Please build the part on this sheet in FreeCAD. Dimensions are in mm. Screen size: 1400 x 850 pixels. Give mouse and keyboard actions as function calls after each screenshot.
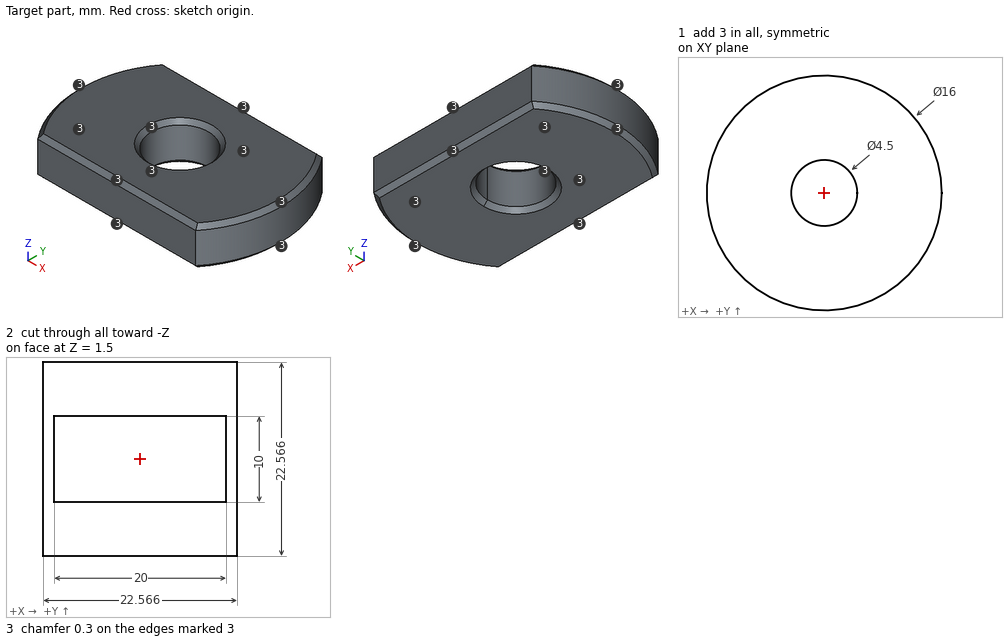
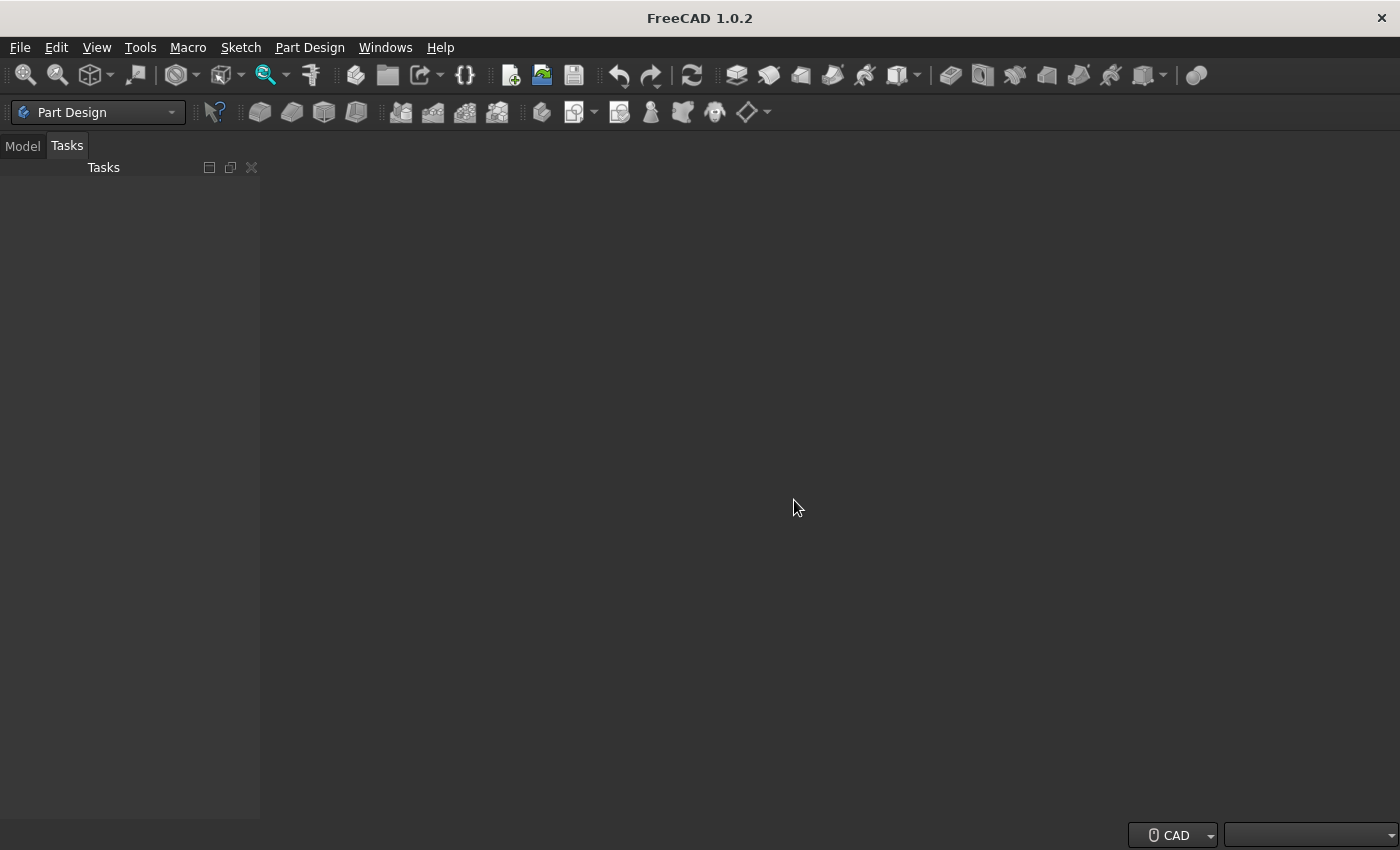
key(ctrl+n)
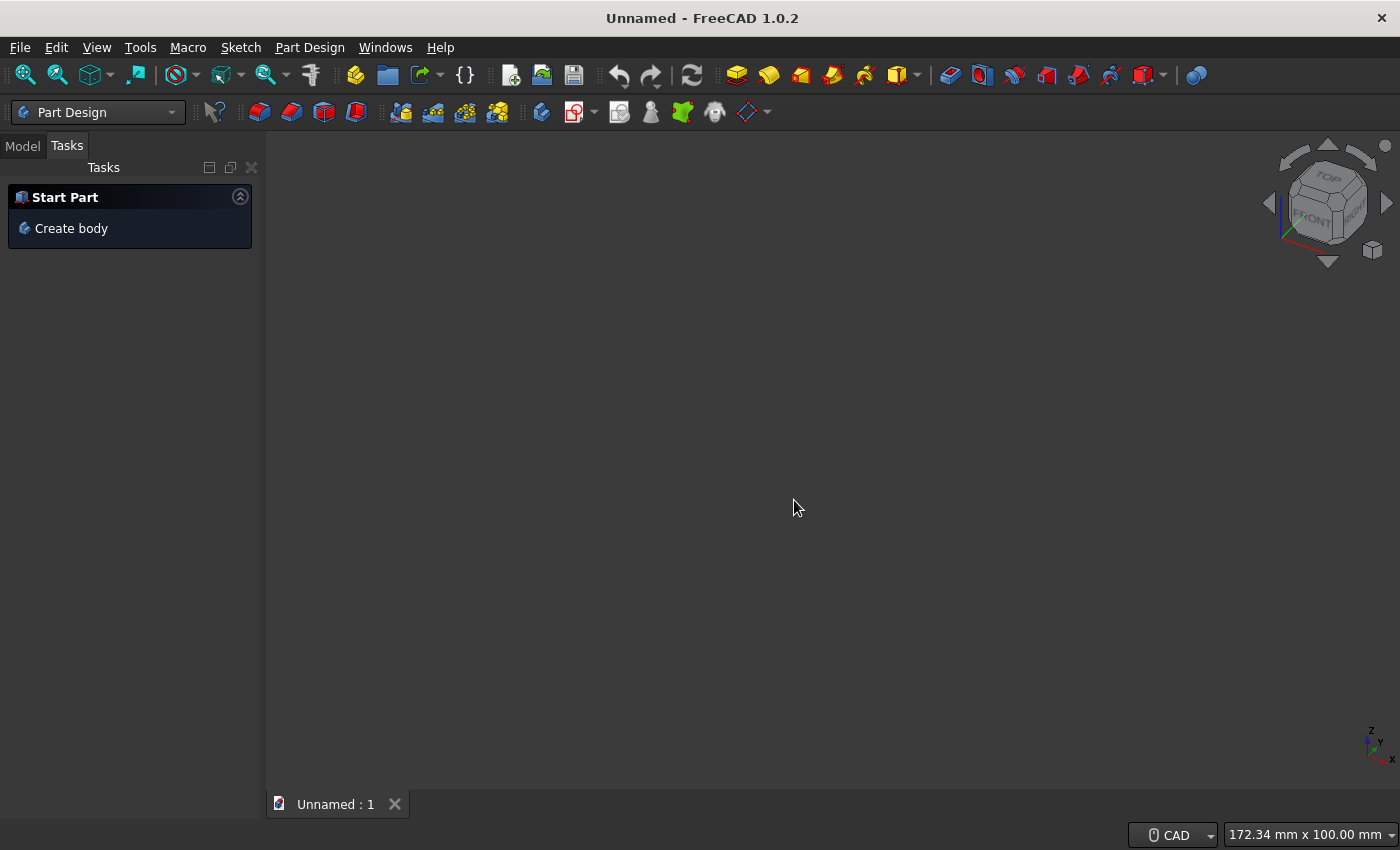
click(574, 112)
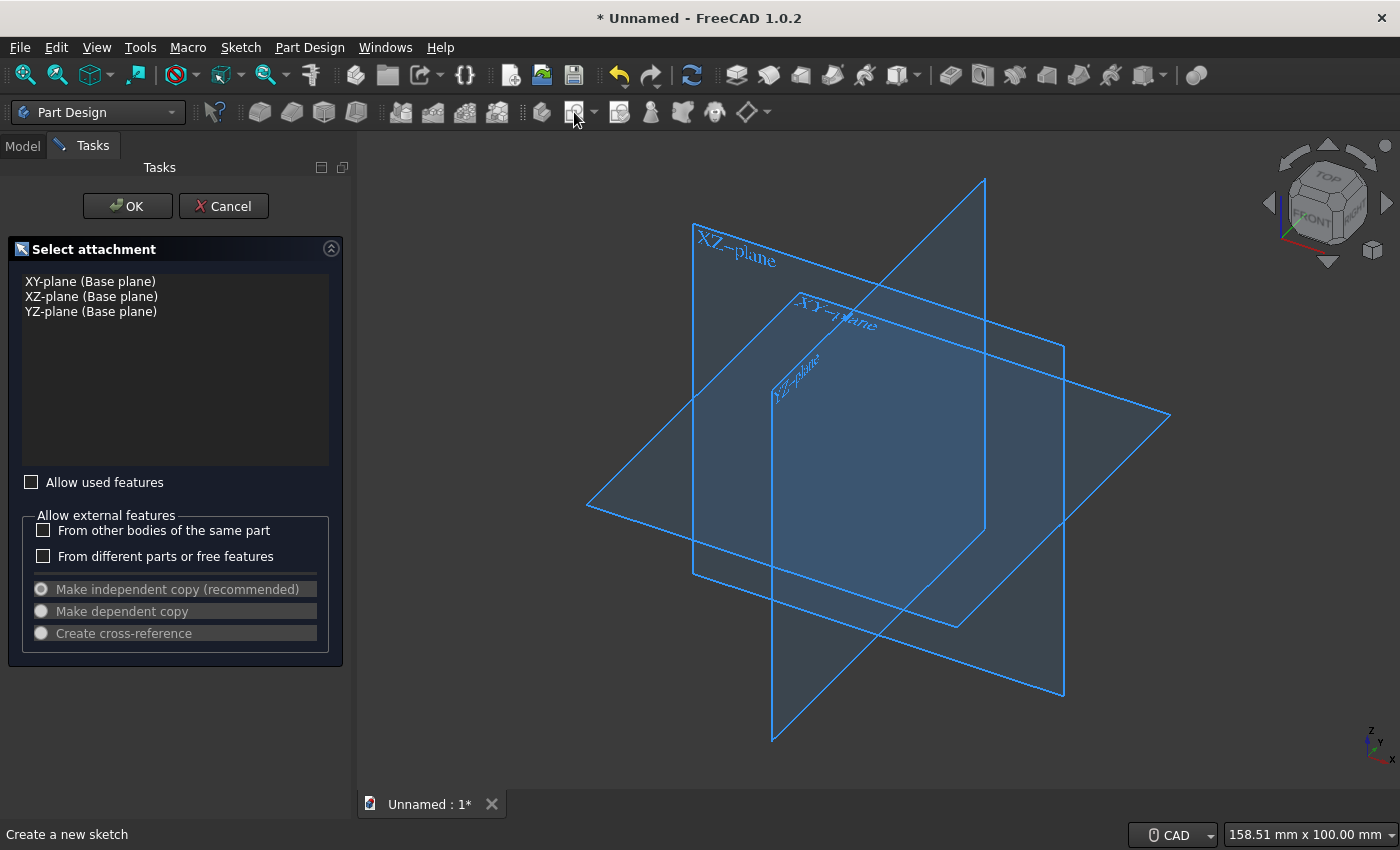
click(82, 282)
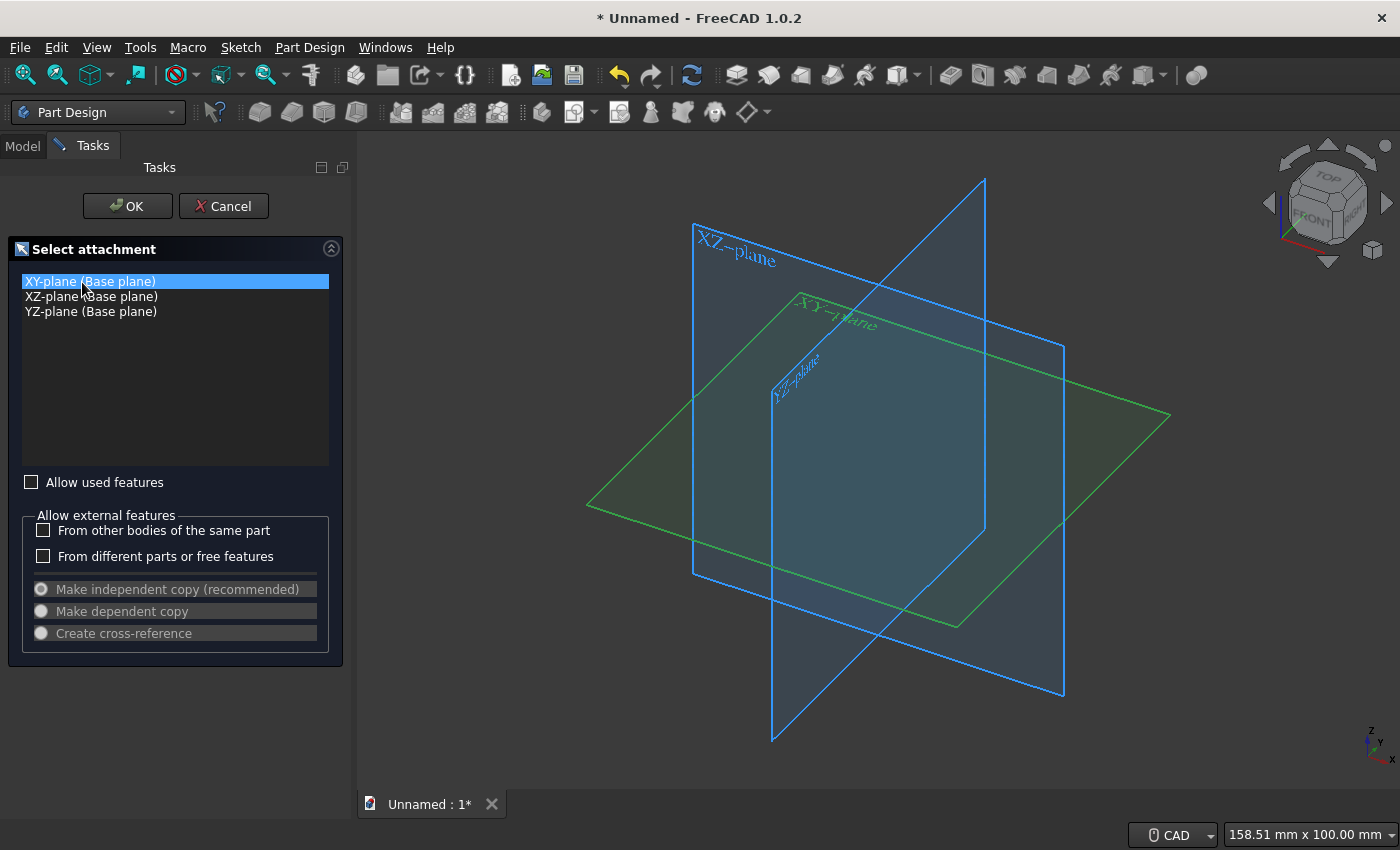
click(128, 206)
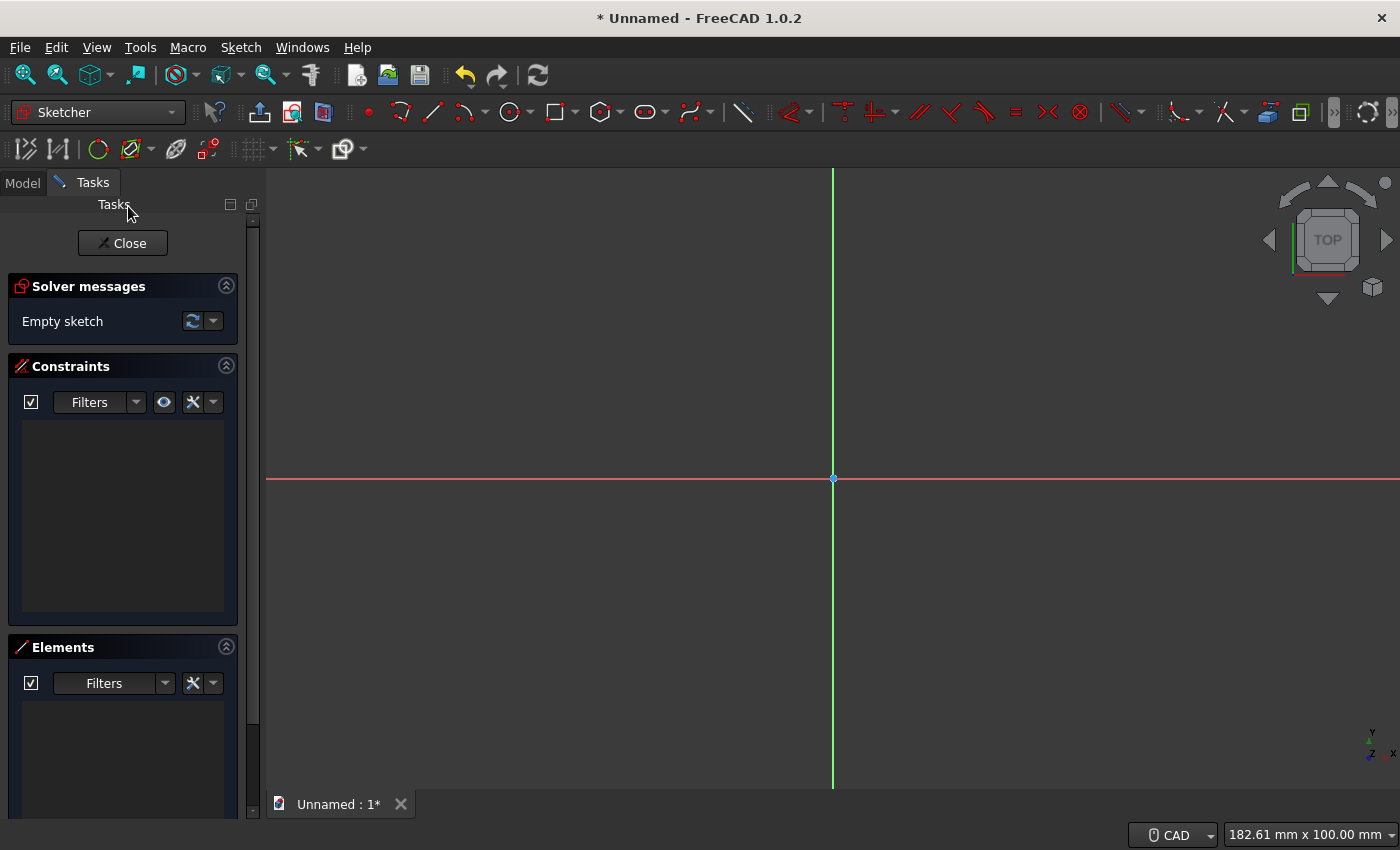
scroll(855, 479, up, 7)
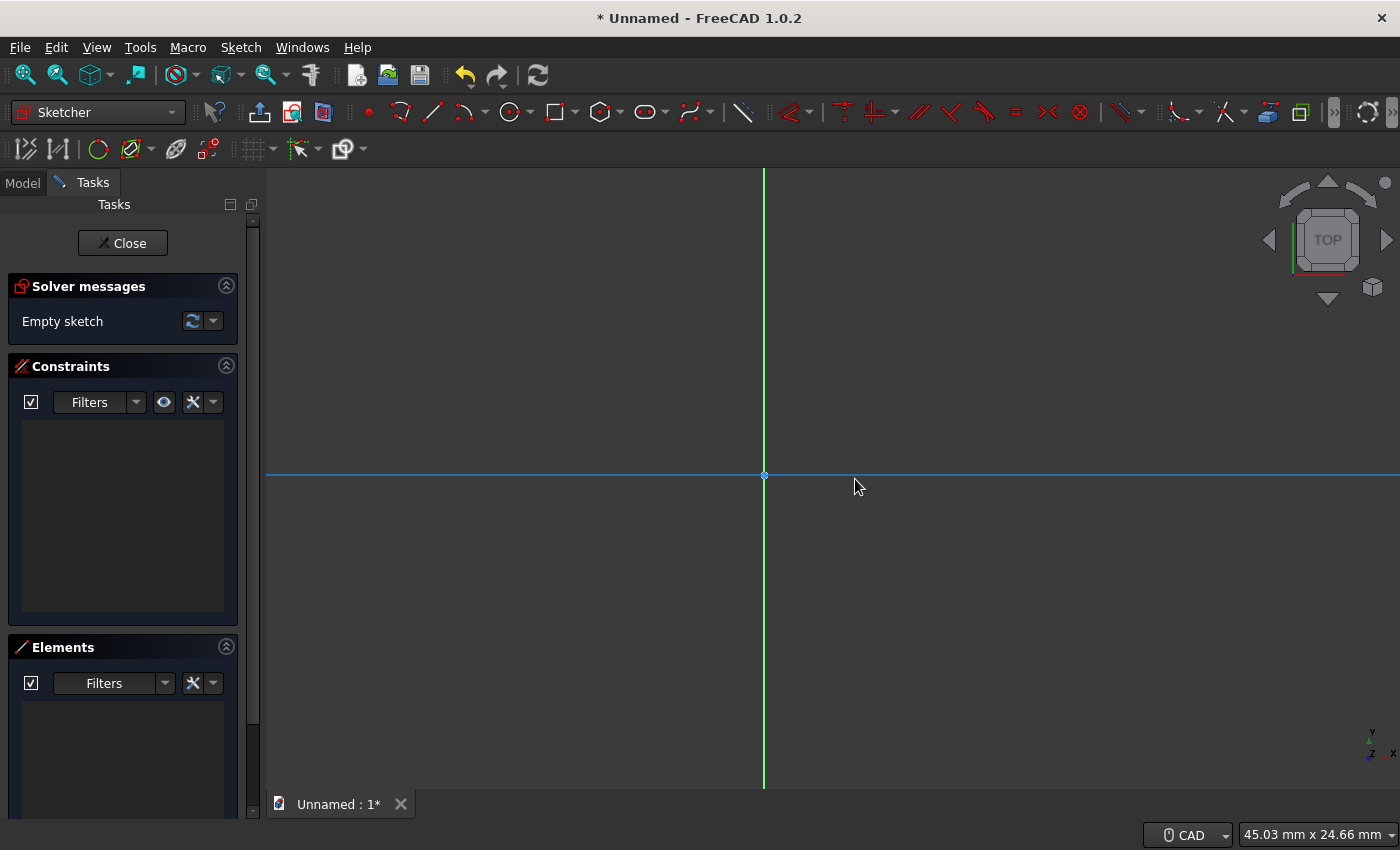
key(g)
key(c)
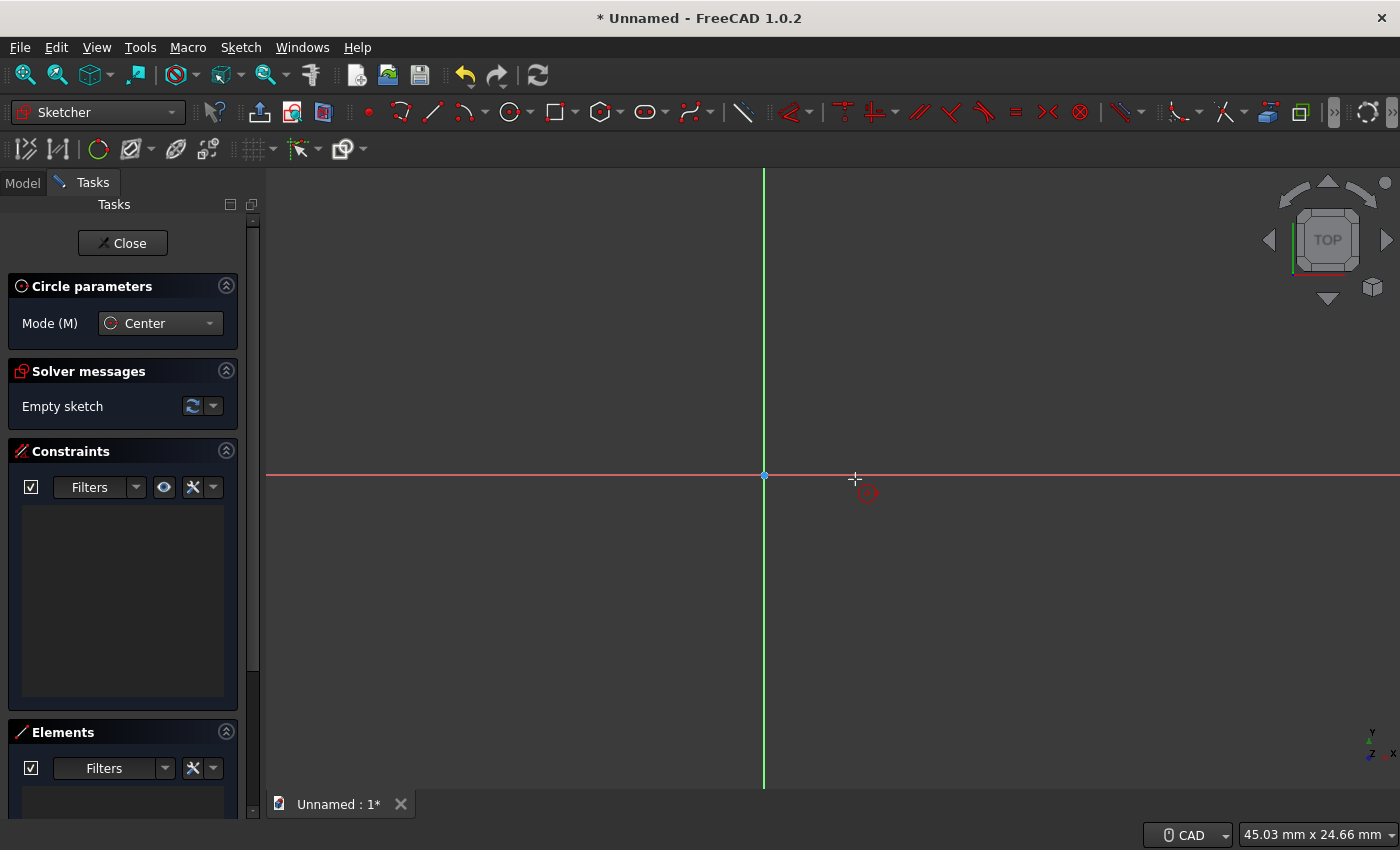
click(764, 475)
click(907, 333)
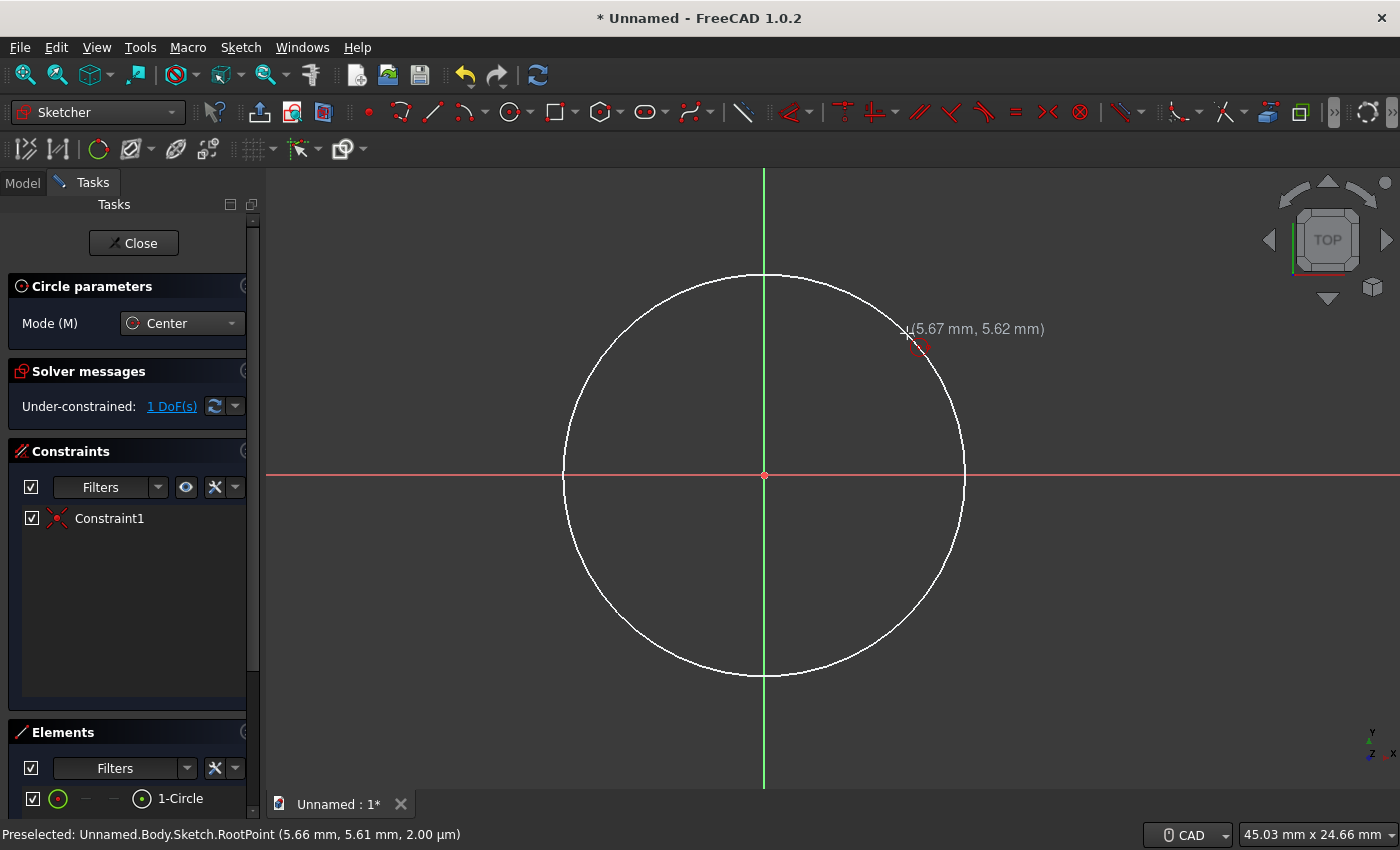
click(764, 475)
click(804, 435)
key(Escape)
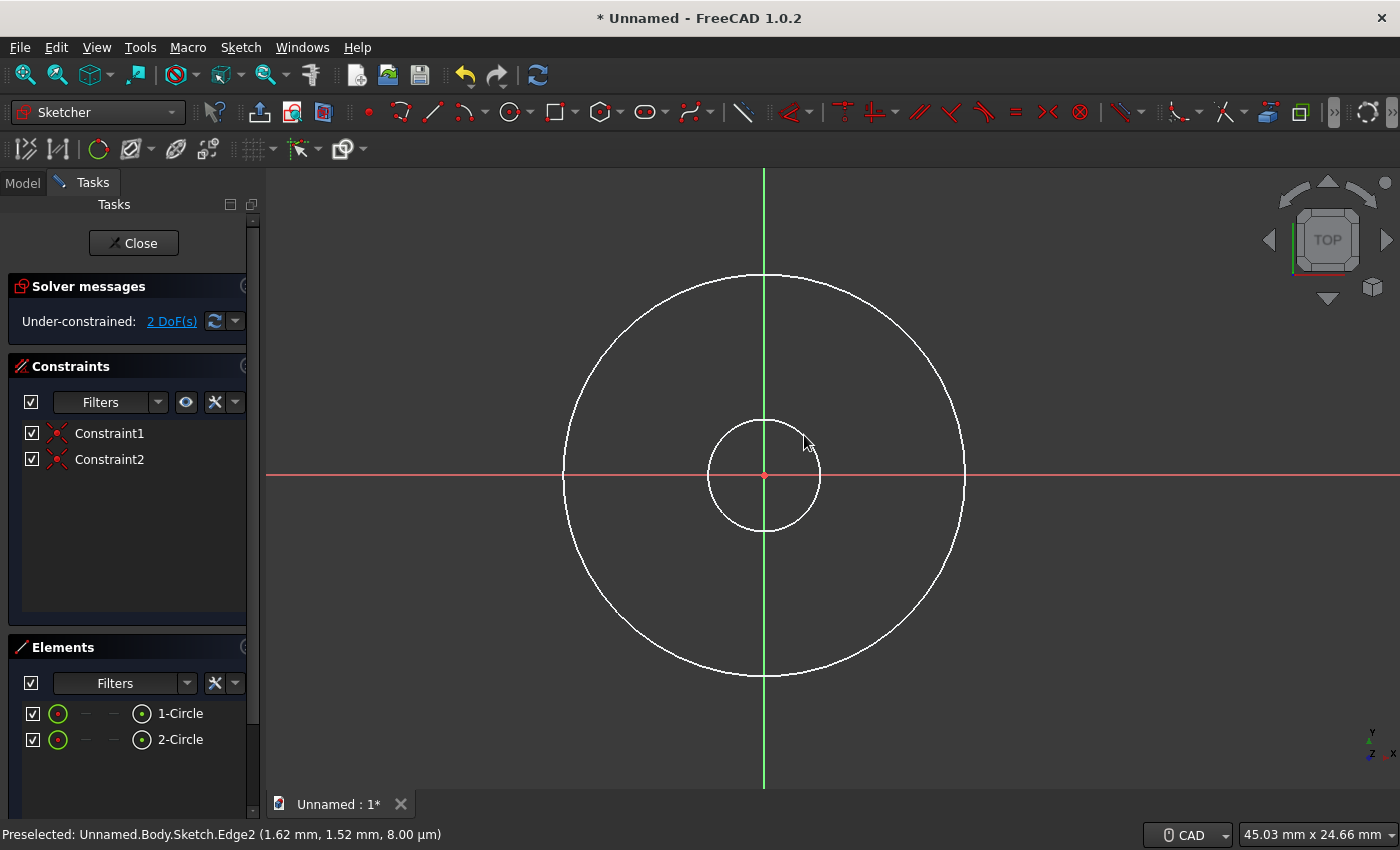
click(906, 333)